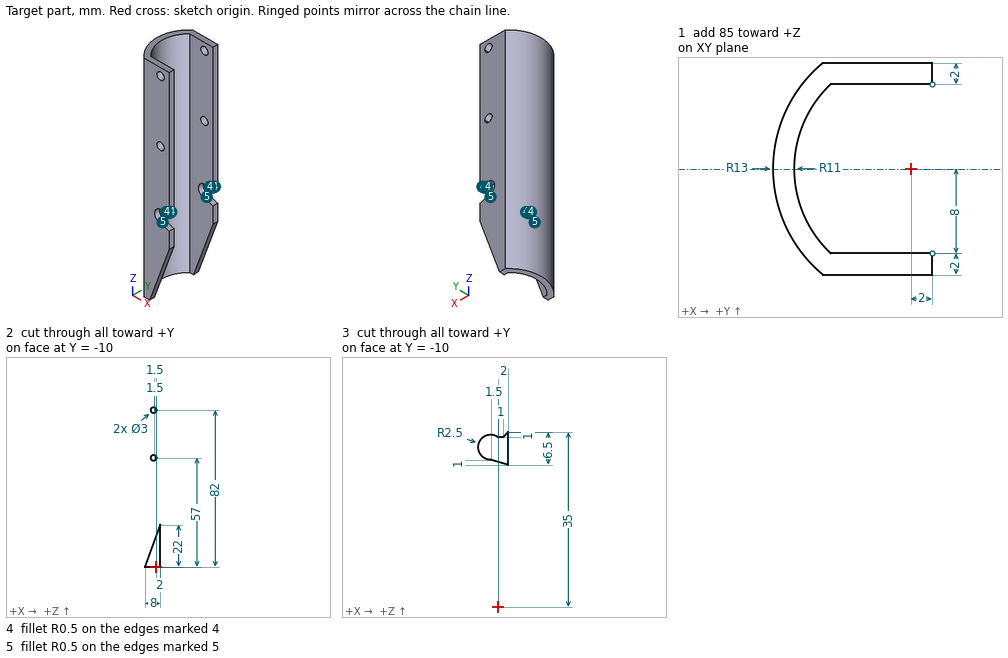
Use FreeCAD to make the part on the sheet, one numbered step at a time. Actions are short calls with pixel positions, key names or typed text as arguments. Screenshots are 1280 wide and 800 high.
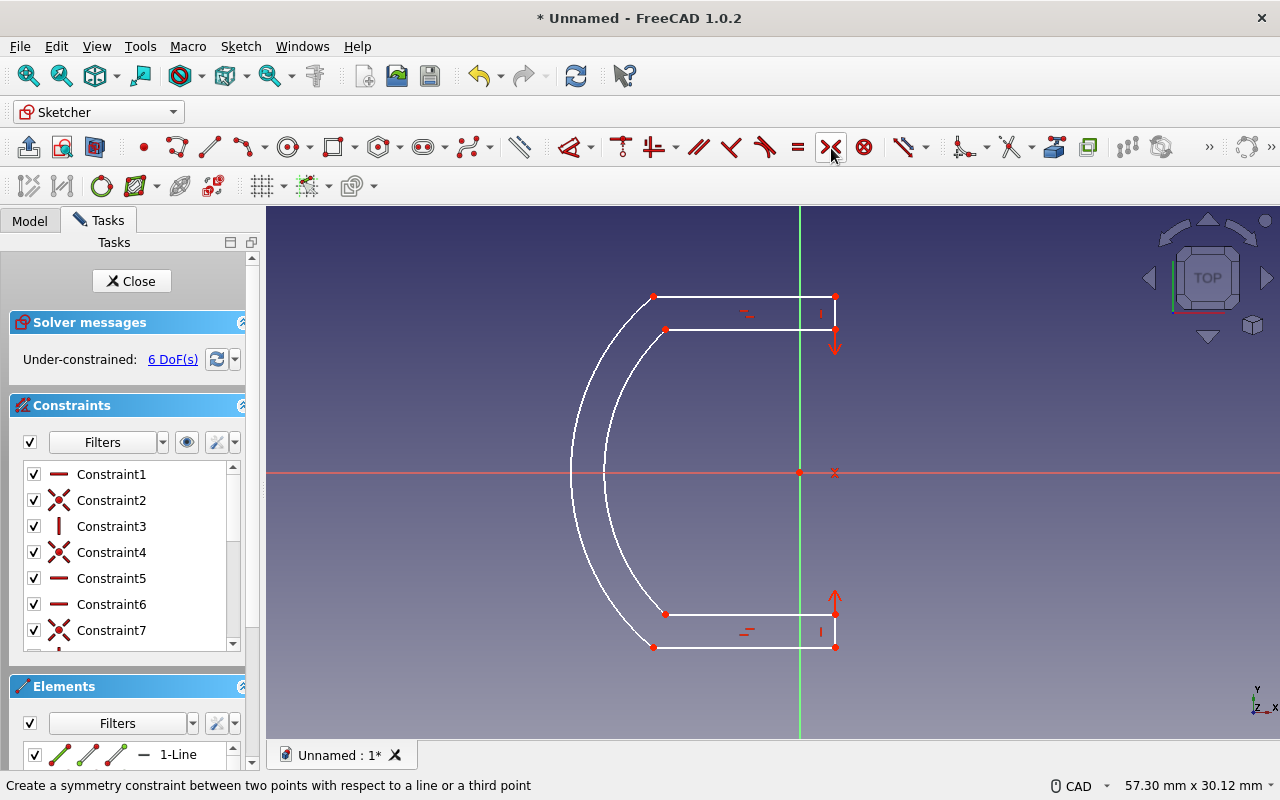
click(568, 148)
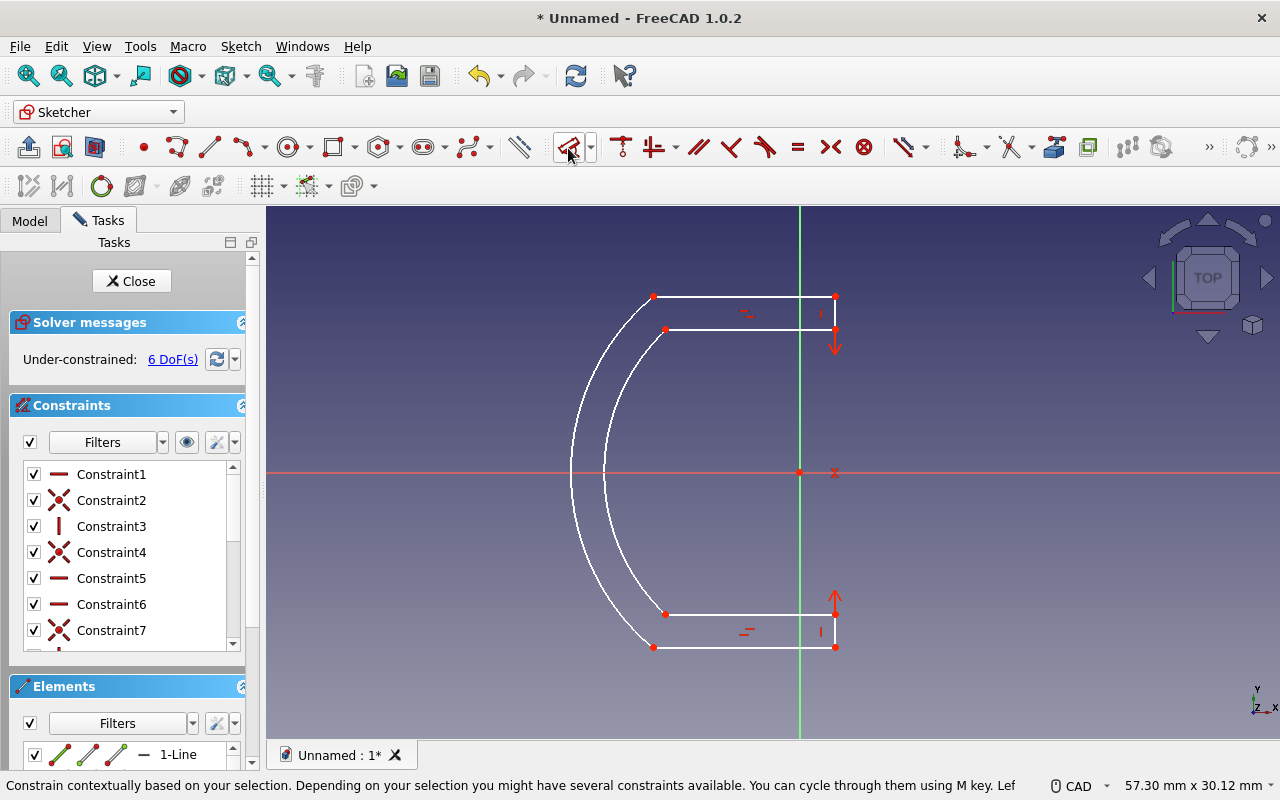
click(615, 410)
click(745, 252)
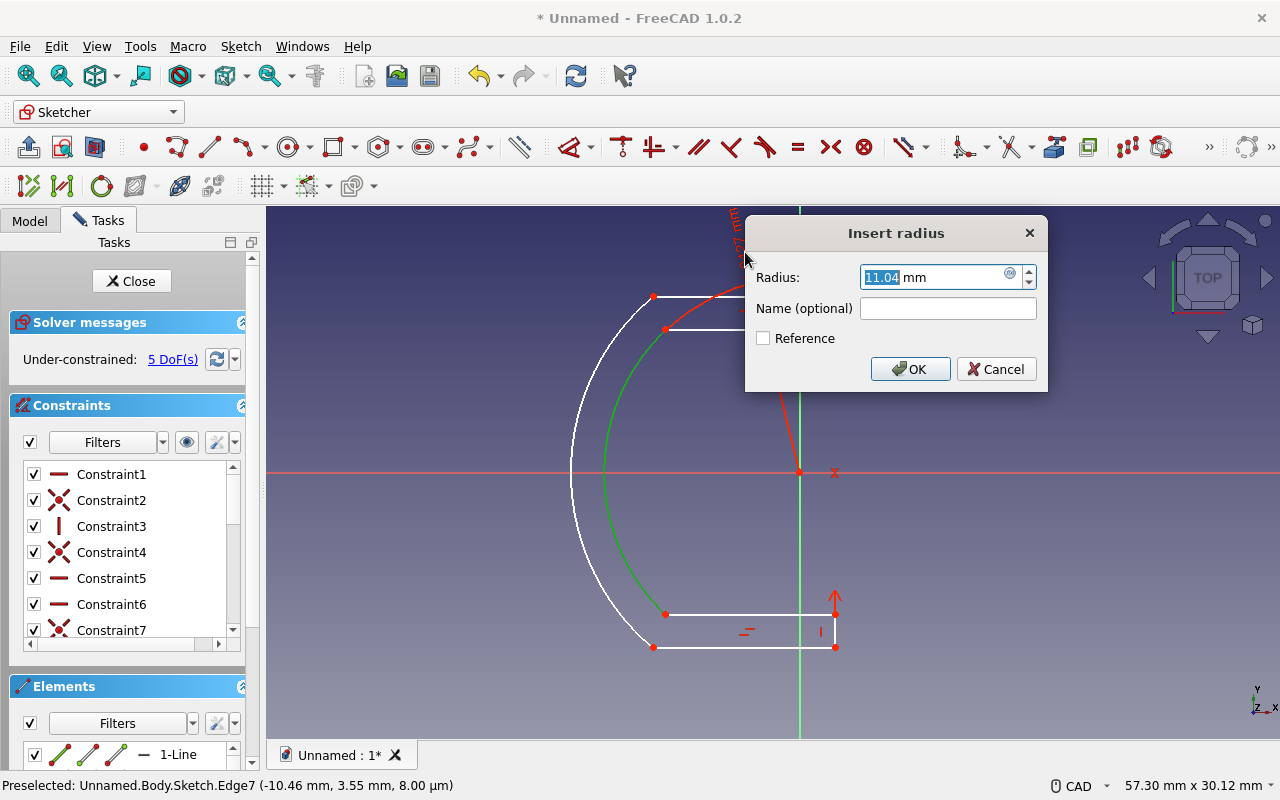
text(11)
key(Return)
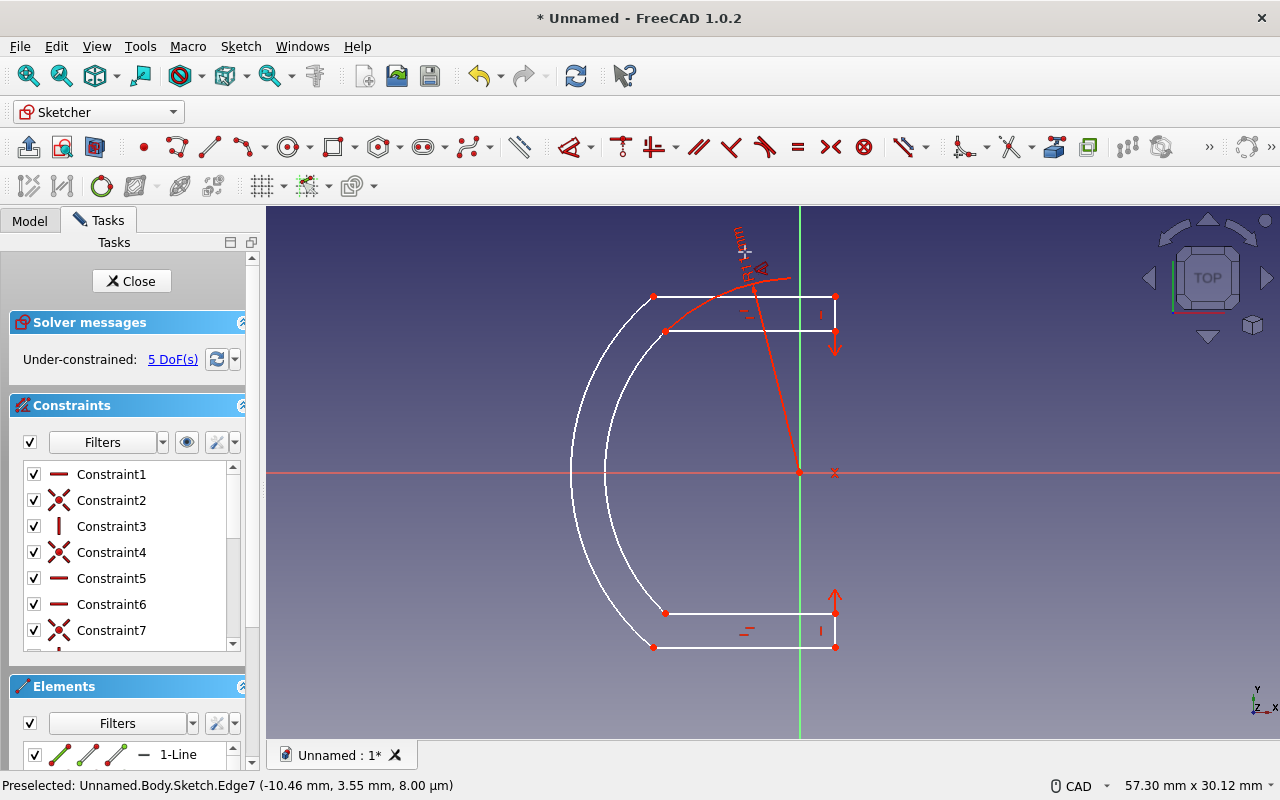
click(585, 394)
click(555, 383)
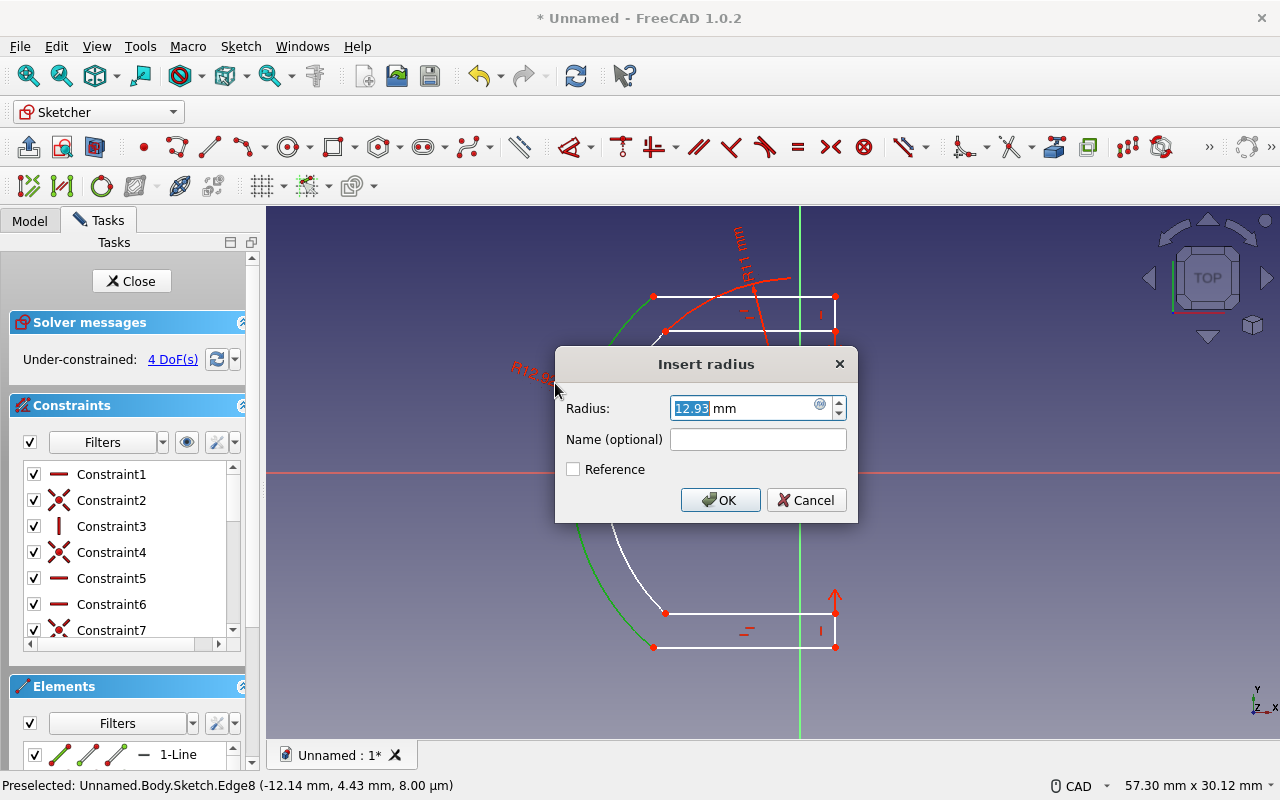
text(13)
key(Return)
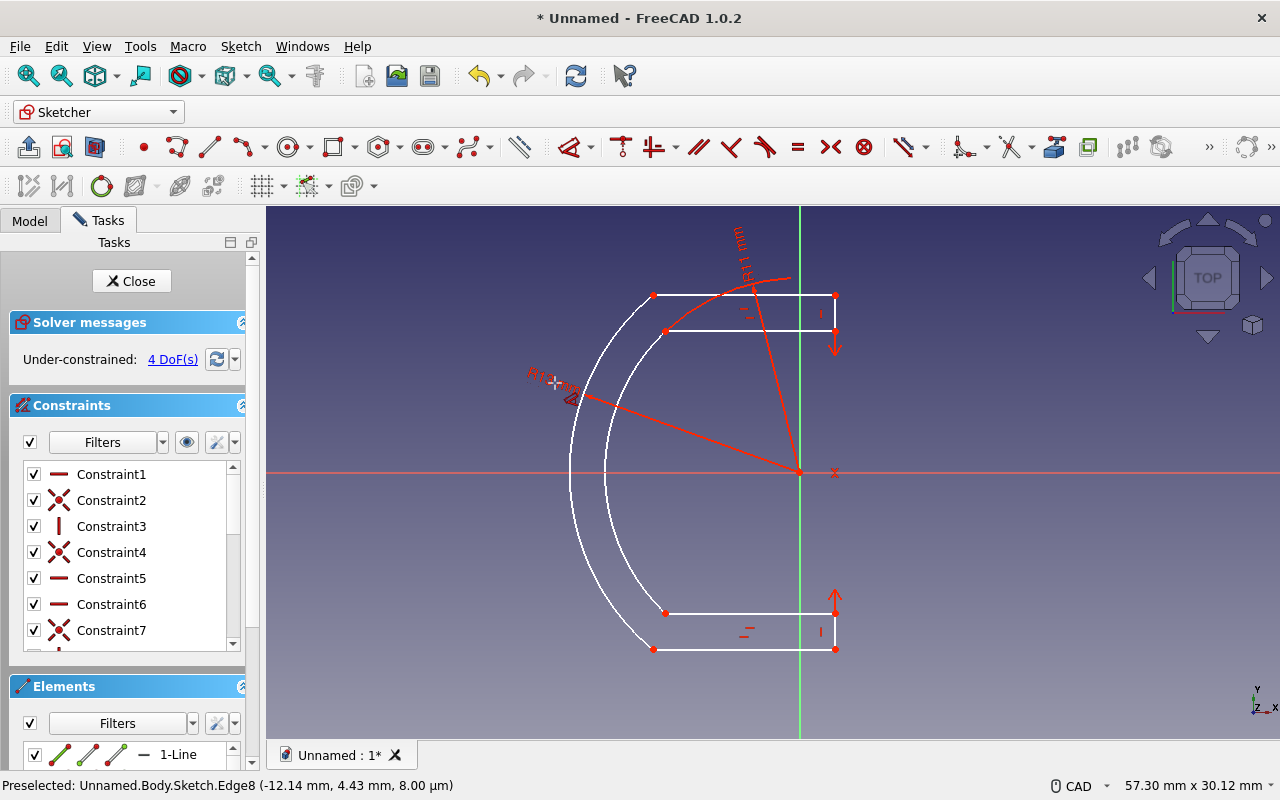
scroll(835, 639, up, 2)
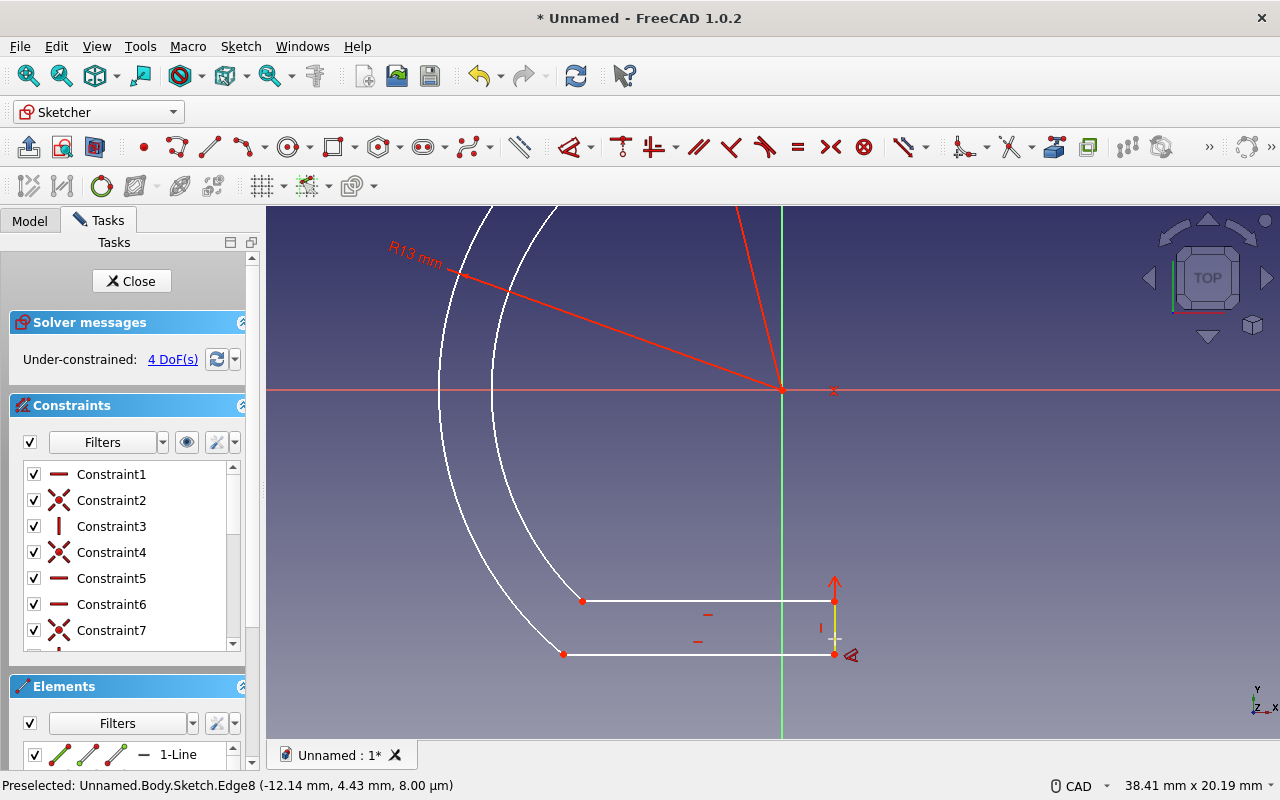
click(835, 639)
click(869, 628)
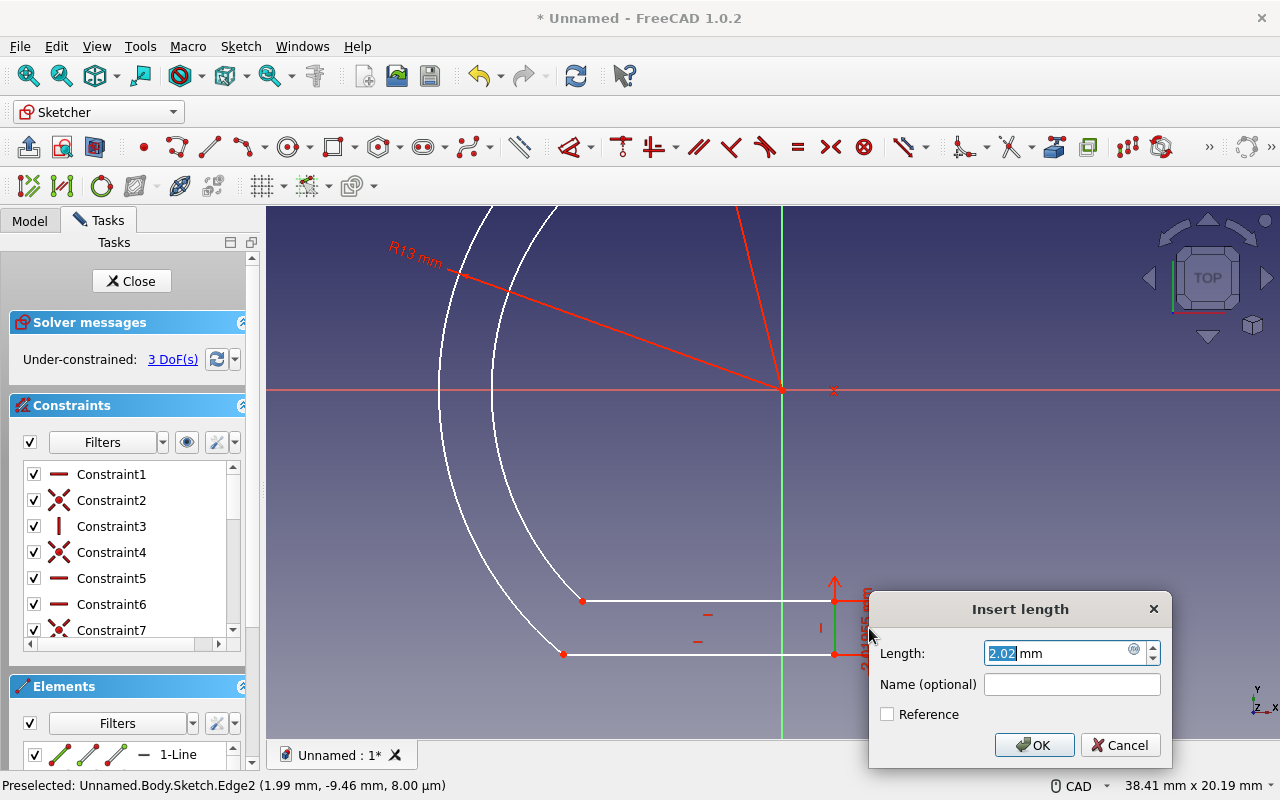
text(2)
key(Return)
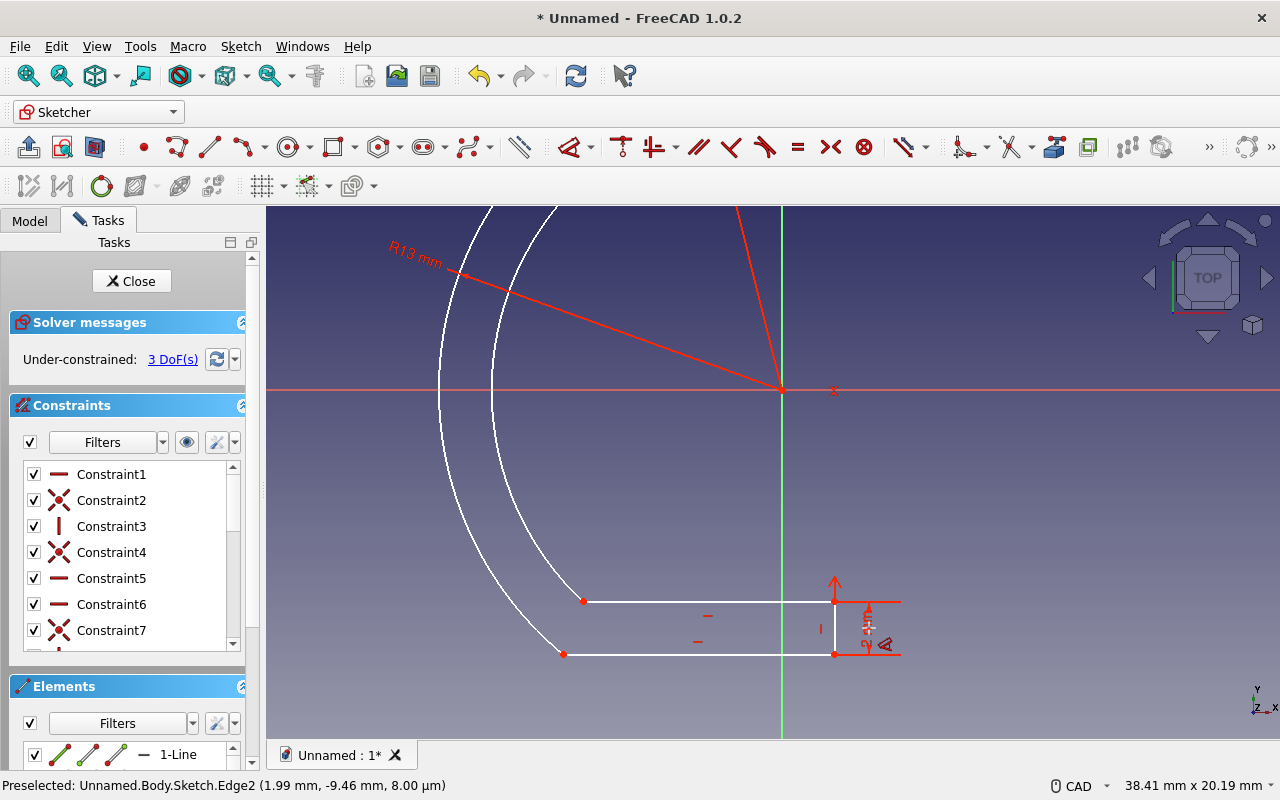
scroll(842, 640, down, 2)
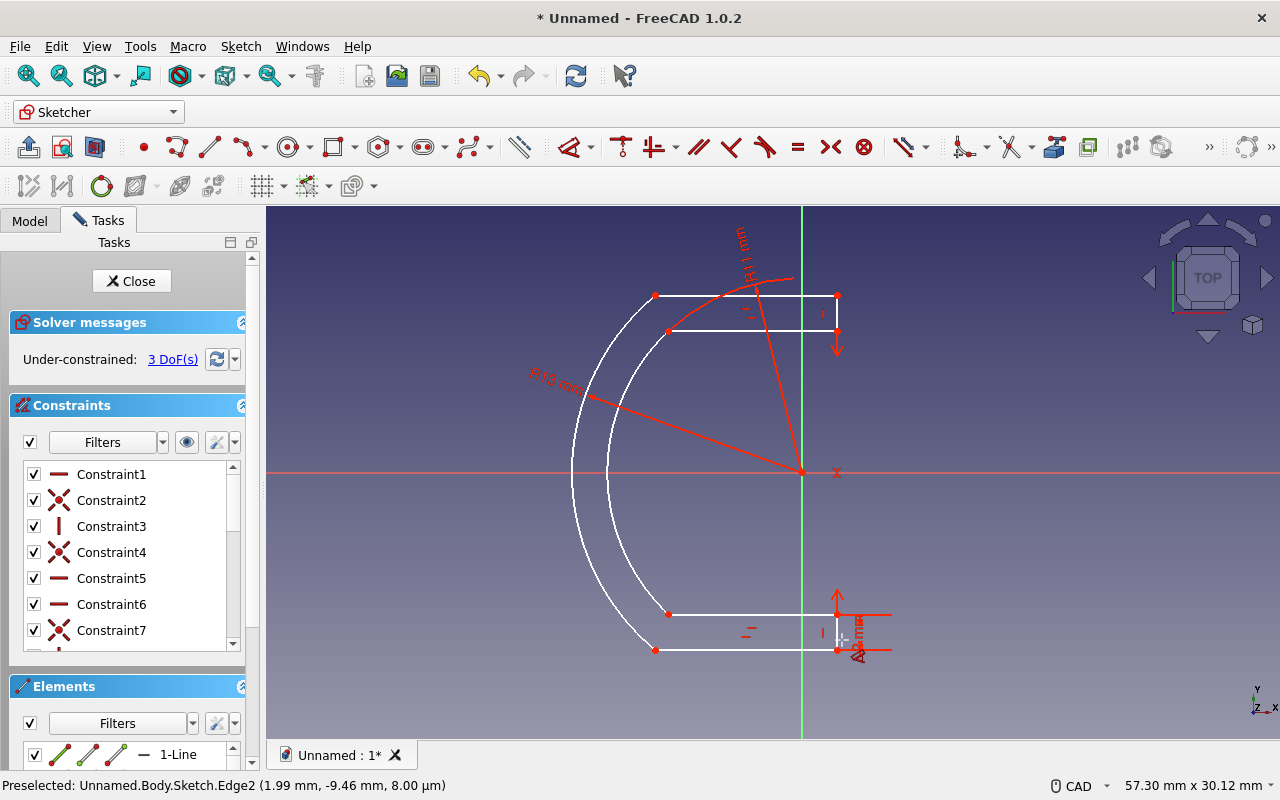
scroll(837, 320, up, 2)